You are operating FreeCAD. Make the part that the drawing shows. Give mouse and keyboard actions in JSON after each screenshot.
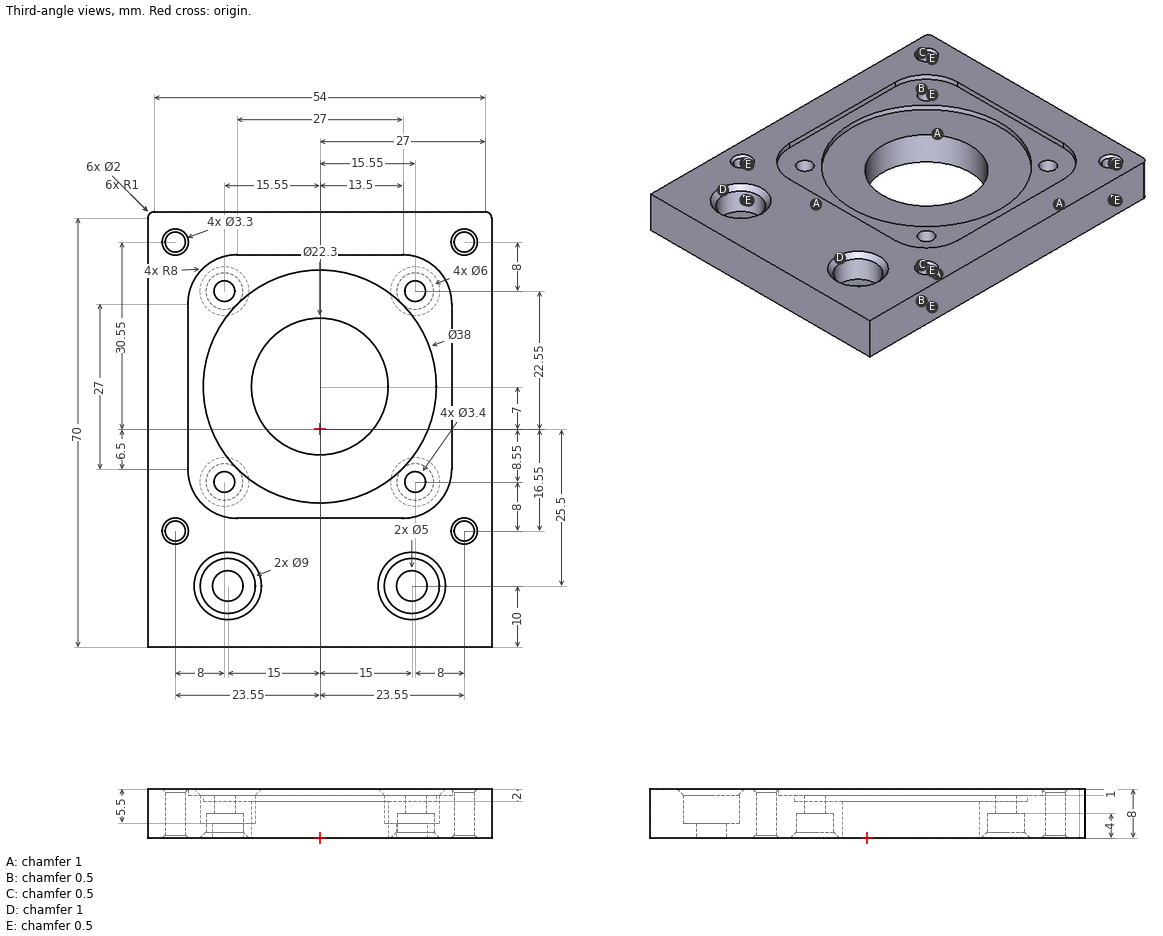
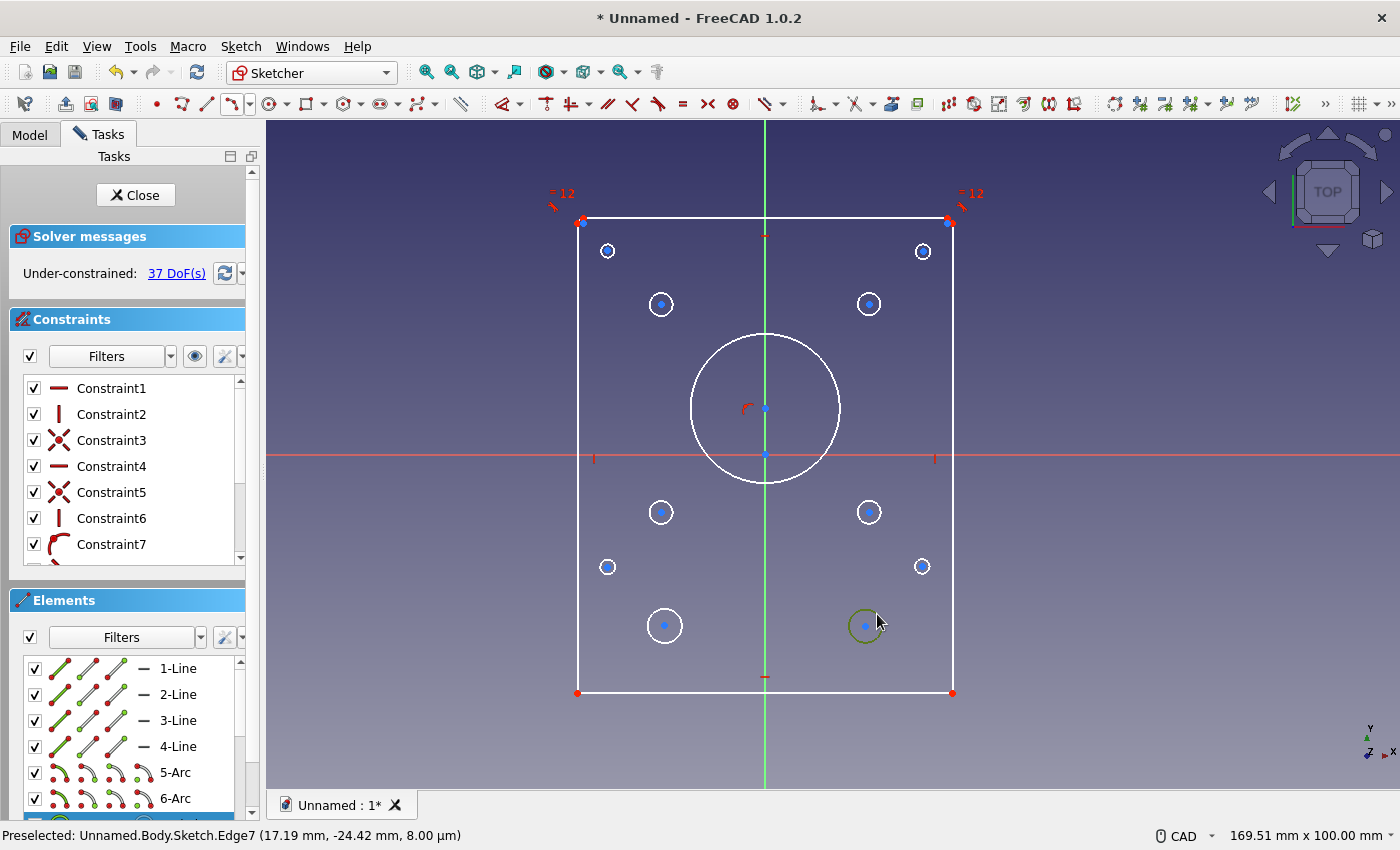
{"action": "left_click", "coordinate": [677, 614]}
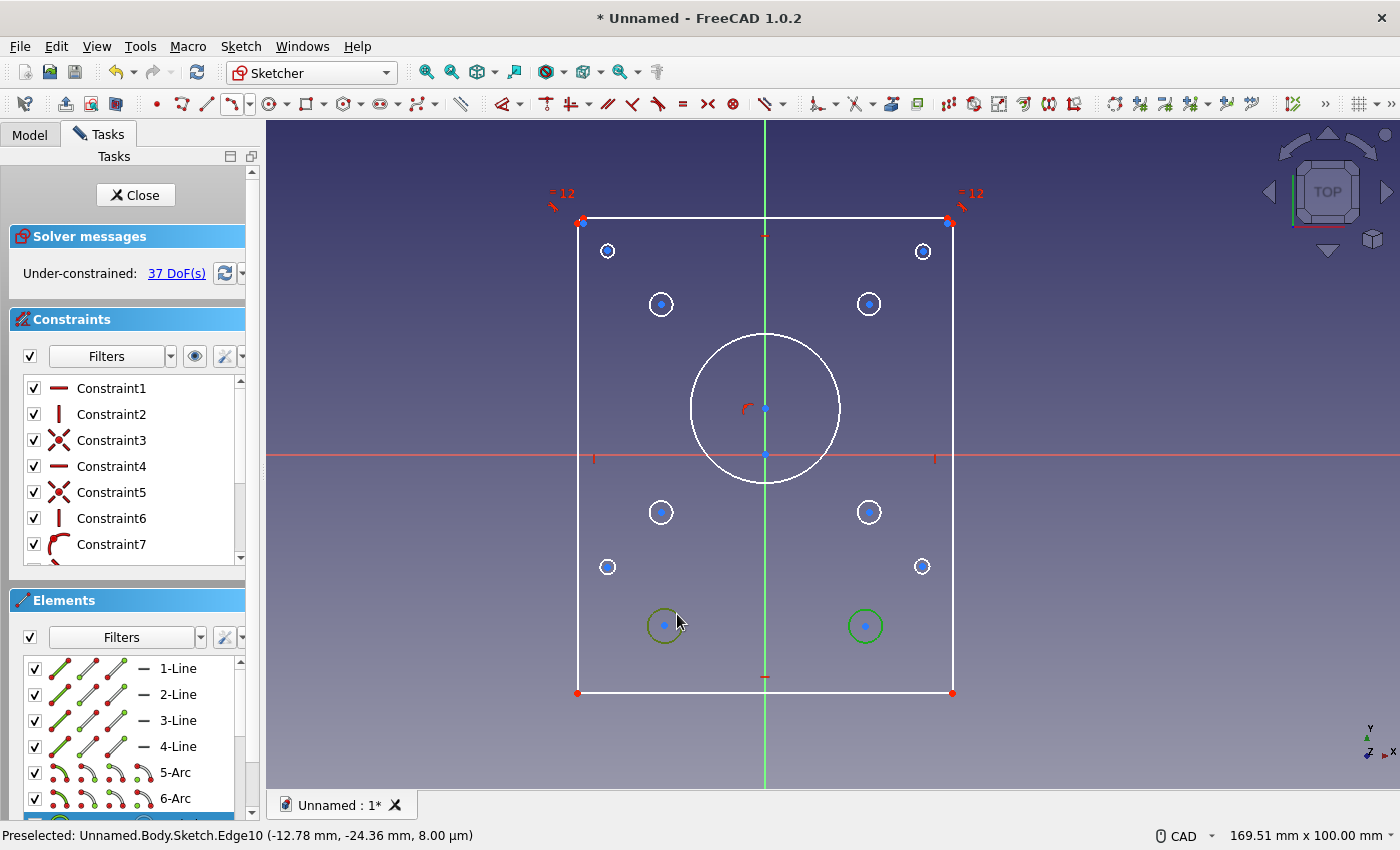
{"action": "key", "text": "e"}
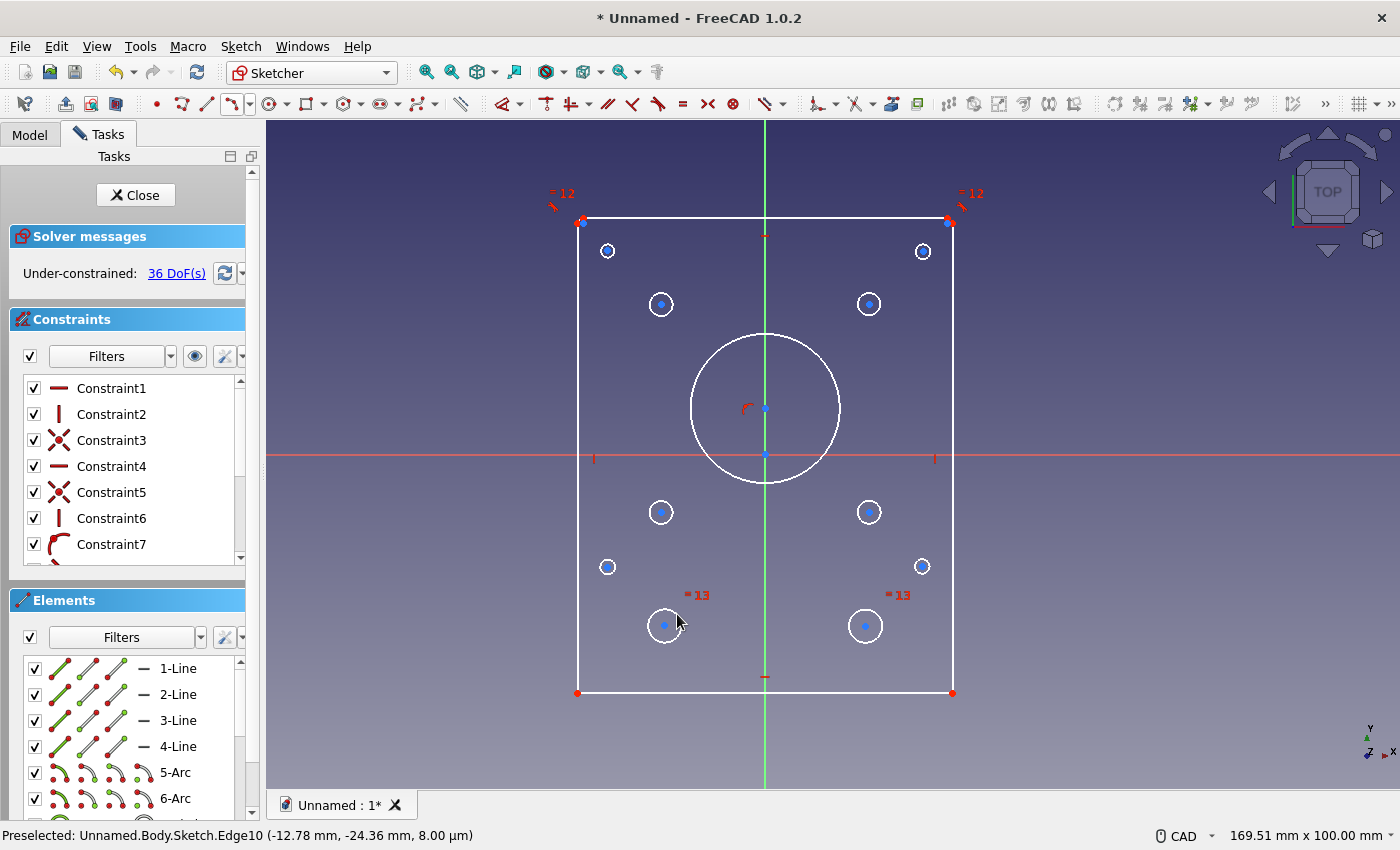
{"action": "scroll", "coordinate": [917, 561], "scroll_direction": "up", "scroll_amount": 4}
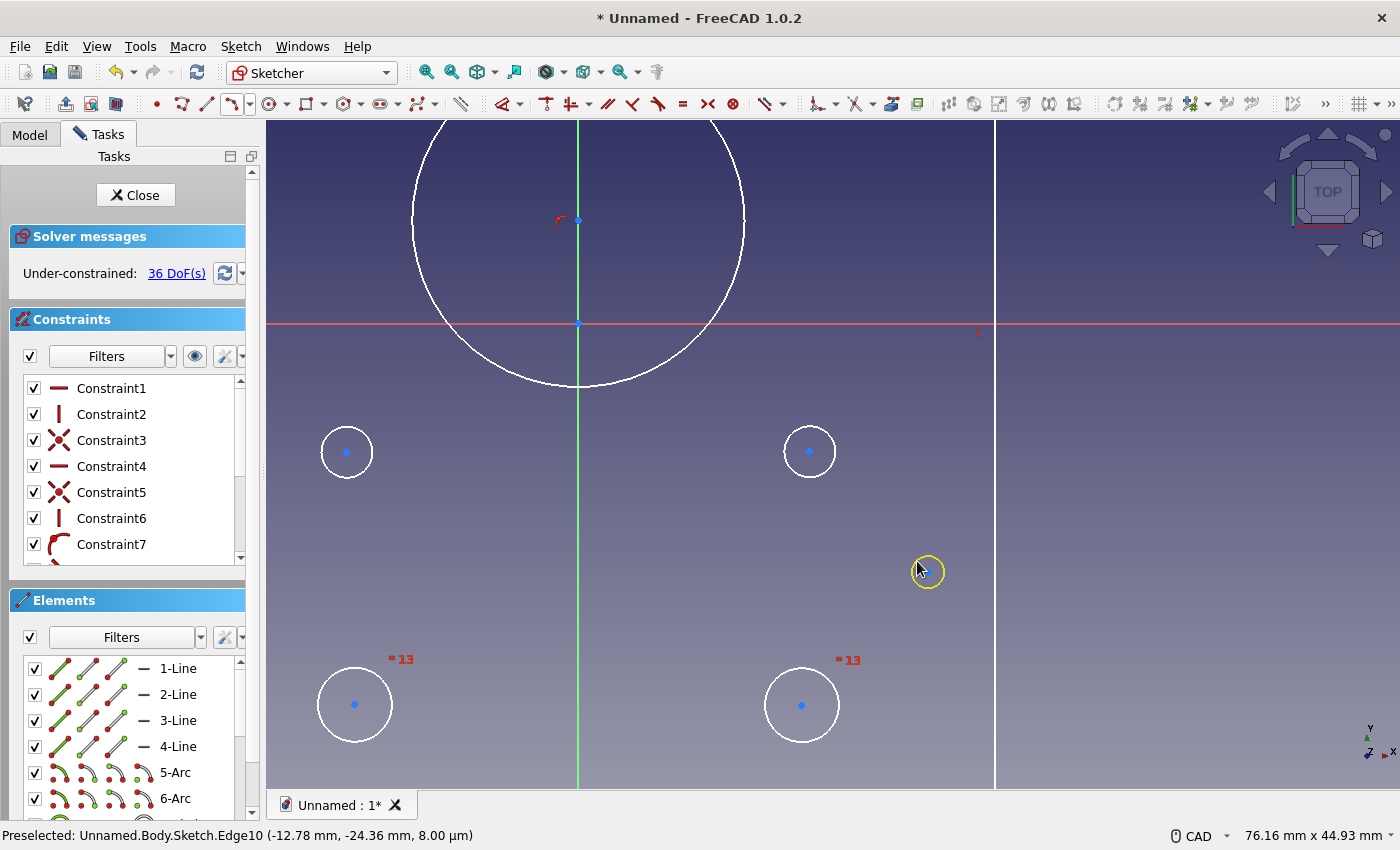
{"action": "left_click", "coordinate": [917, 561]}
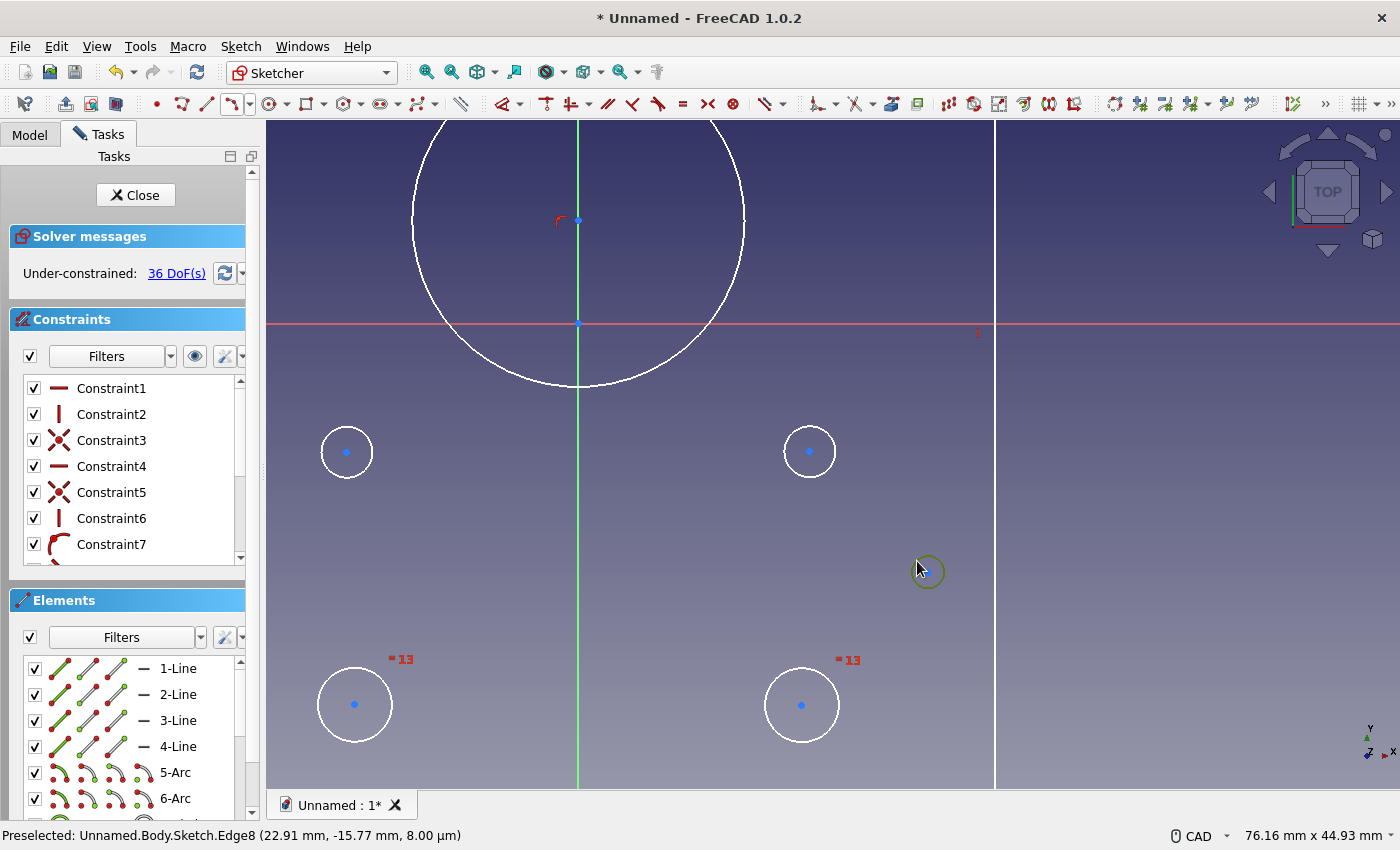
{"action": "scroll", "coordinate": [916, 561], "scroll_direction": "down", "scroll_amount": 4}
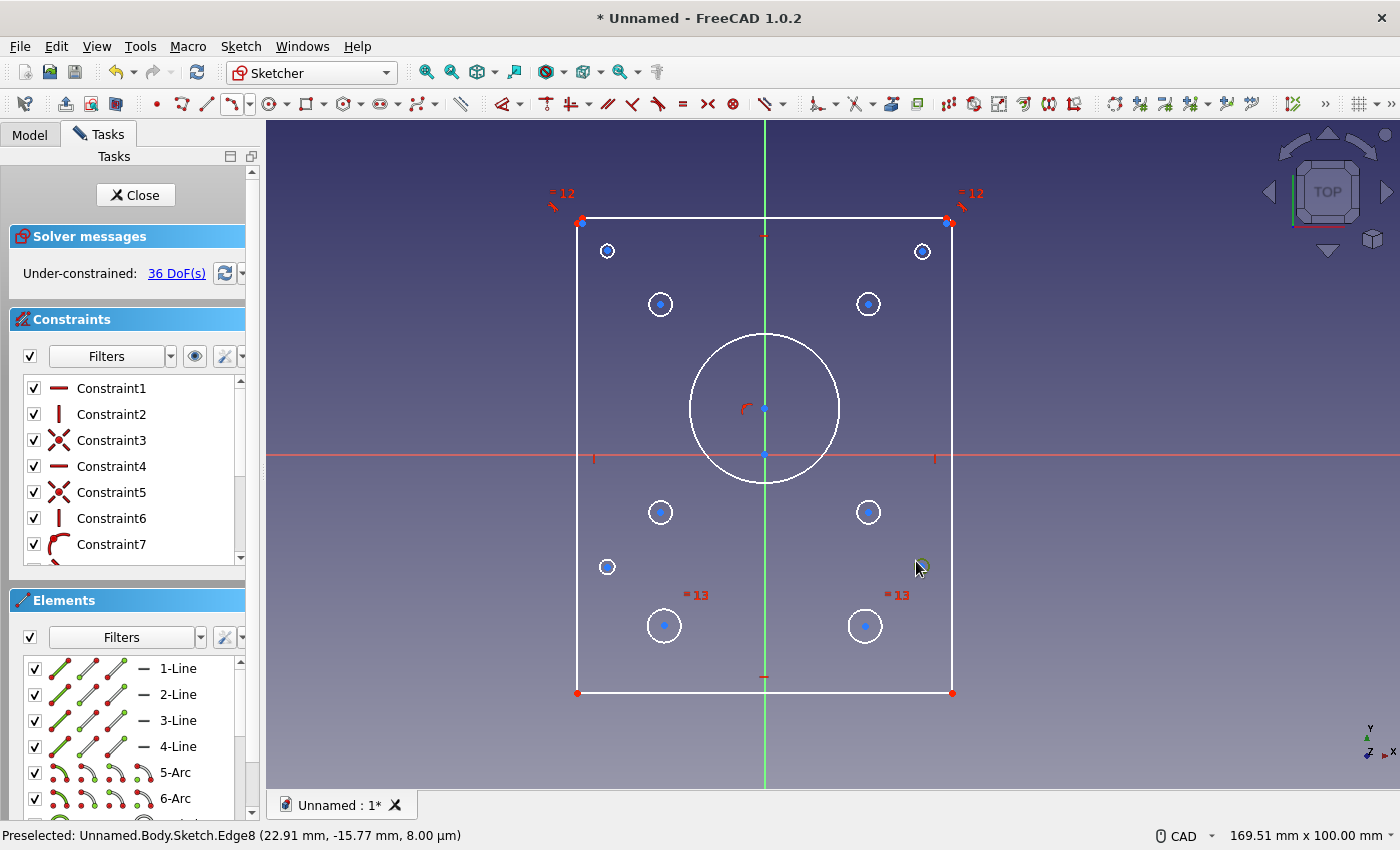
{"action": "scroll", "coordinate": [612, 562], "scroll_direction": "up", "scroll_amount": 4}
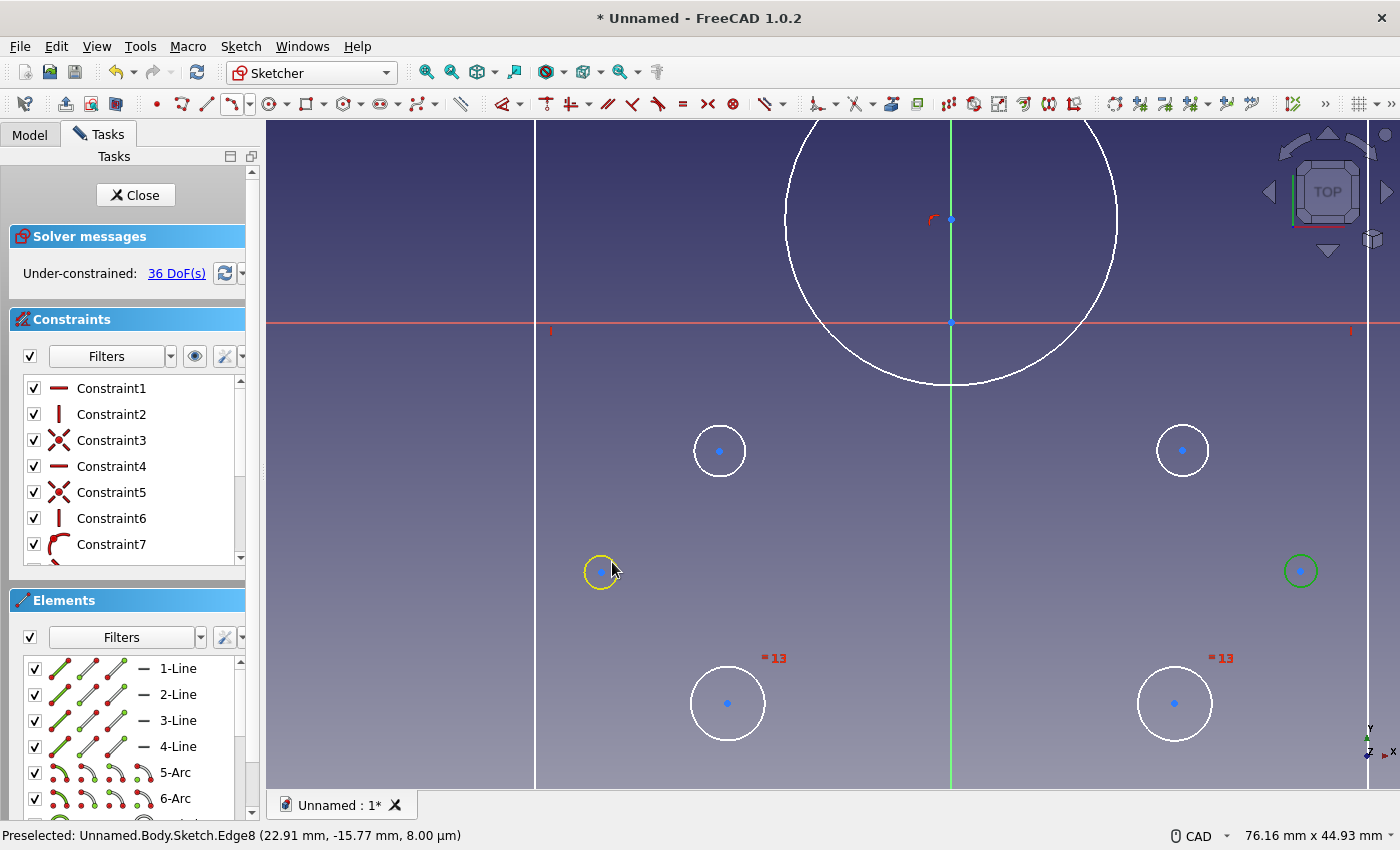
{"action": "left_click", "coordinate": [613, 561]}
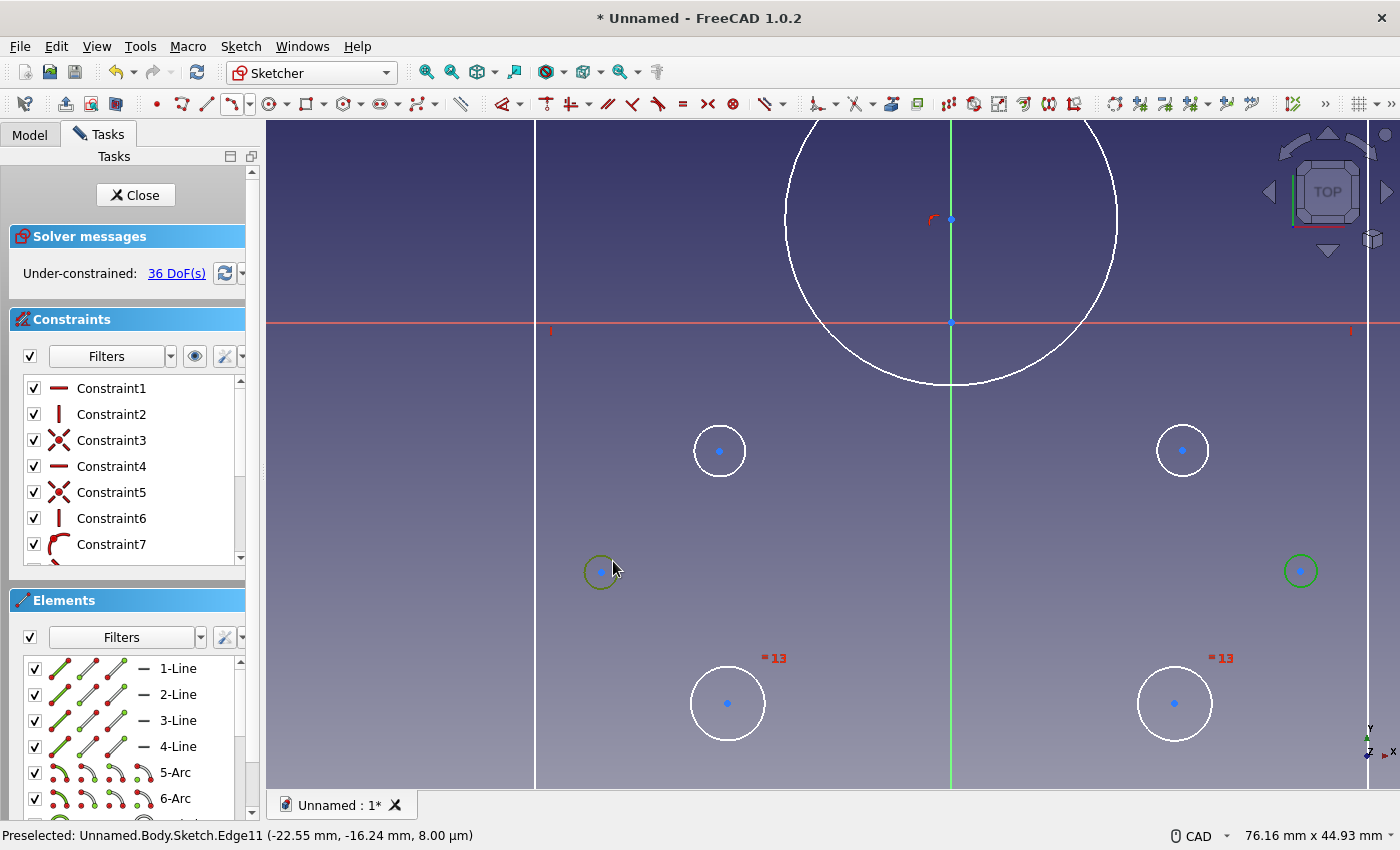
{"action": "scroll", "coordinate": [612, 562], "scroll_direction": "down", "scroll_amount": 4}